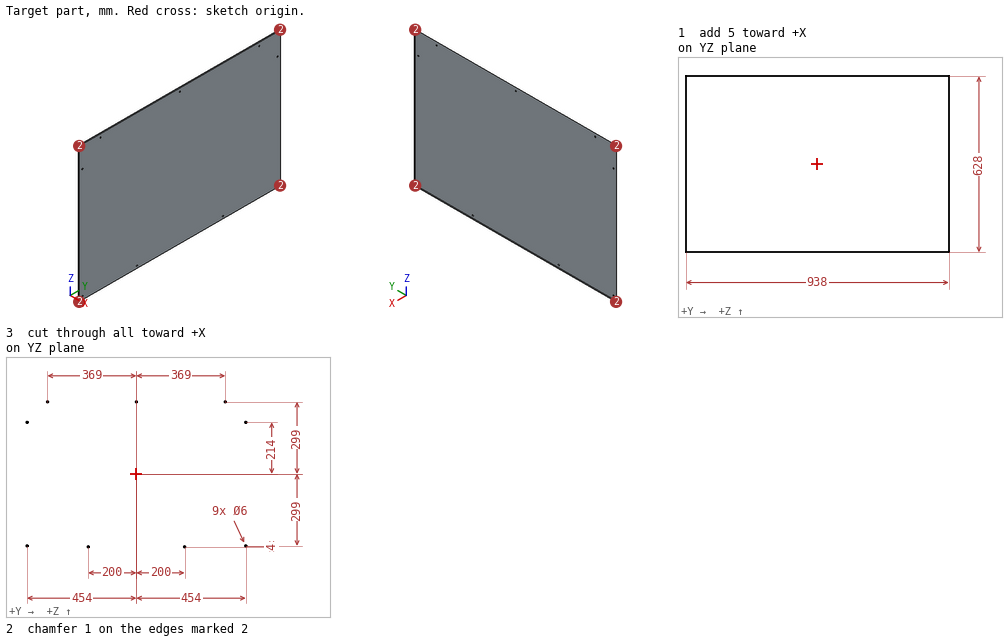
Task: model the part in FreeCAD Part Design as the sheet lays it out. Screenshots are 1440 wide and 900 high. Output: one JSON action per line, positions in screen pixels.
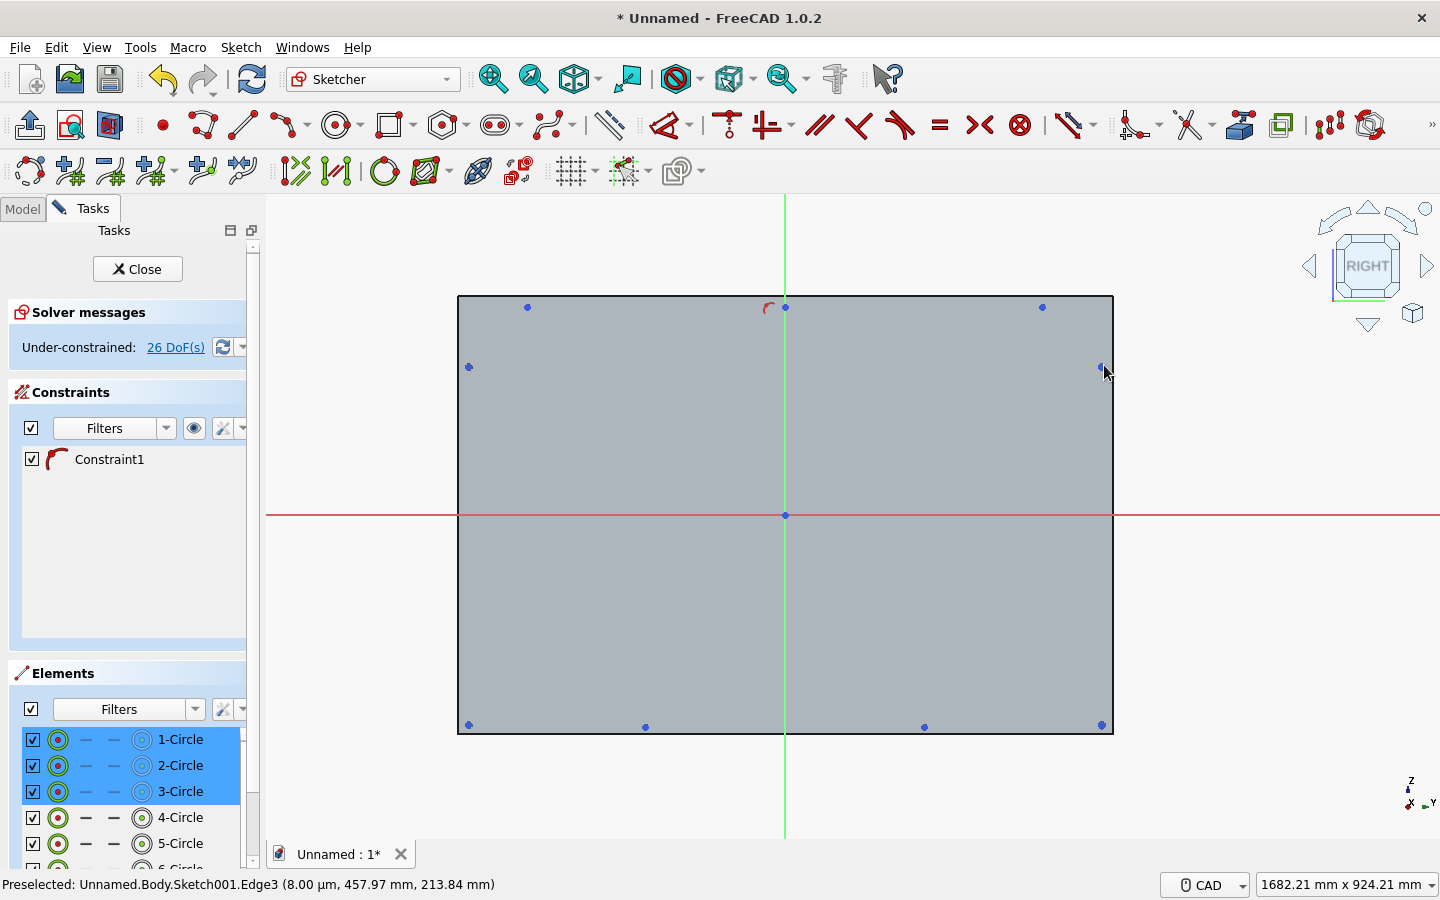
{"action": "scroll", "coordinate": [1045, 305], "scroll_direction": "up", "scroll_amount": 9}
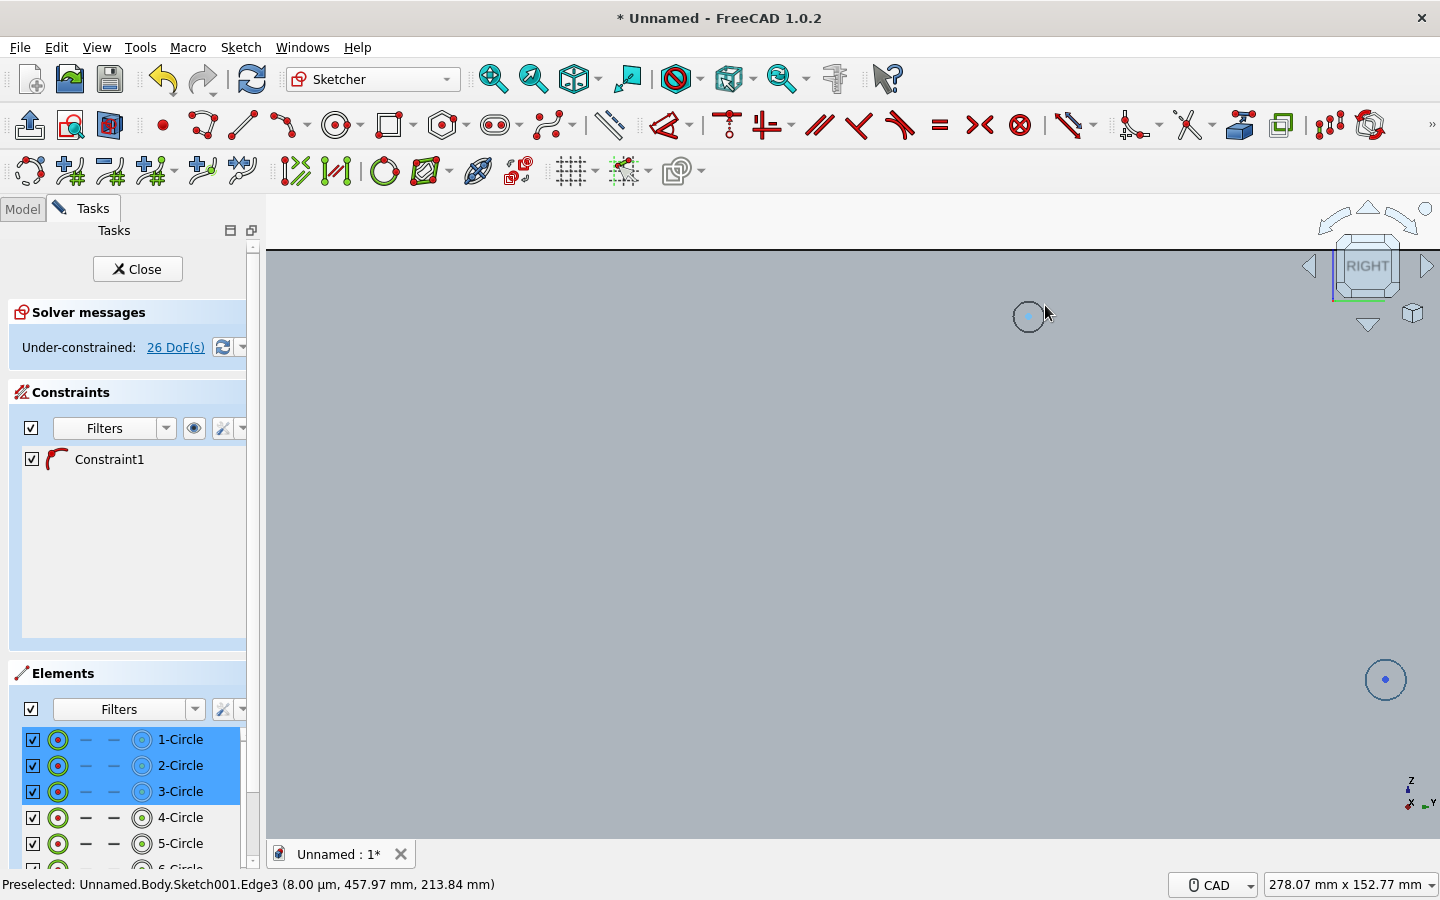
{"action": "left_click", "coordinate": [1040, 306]}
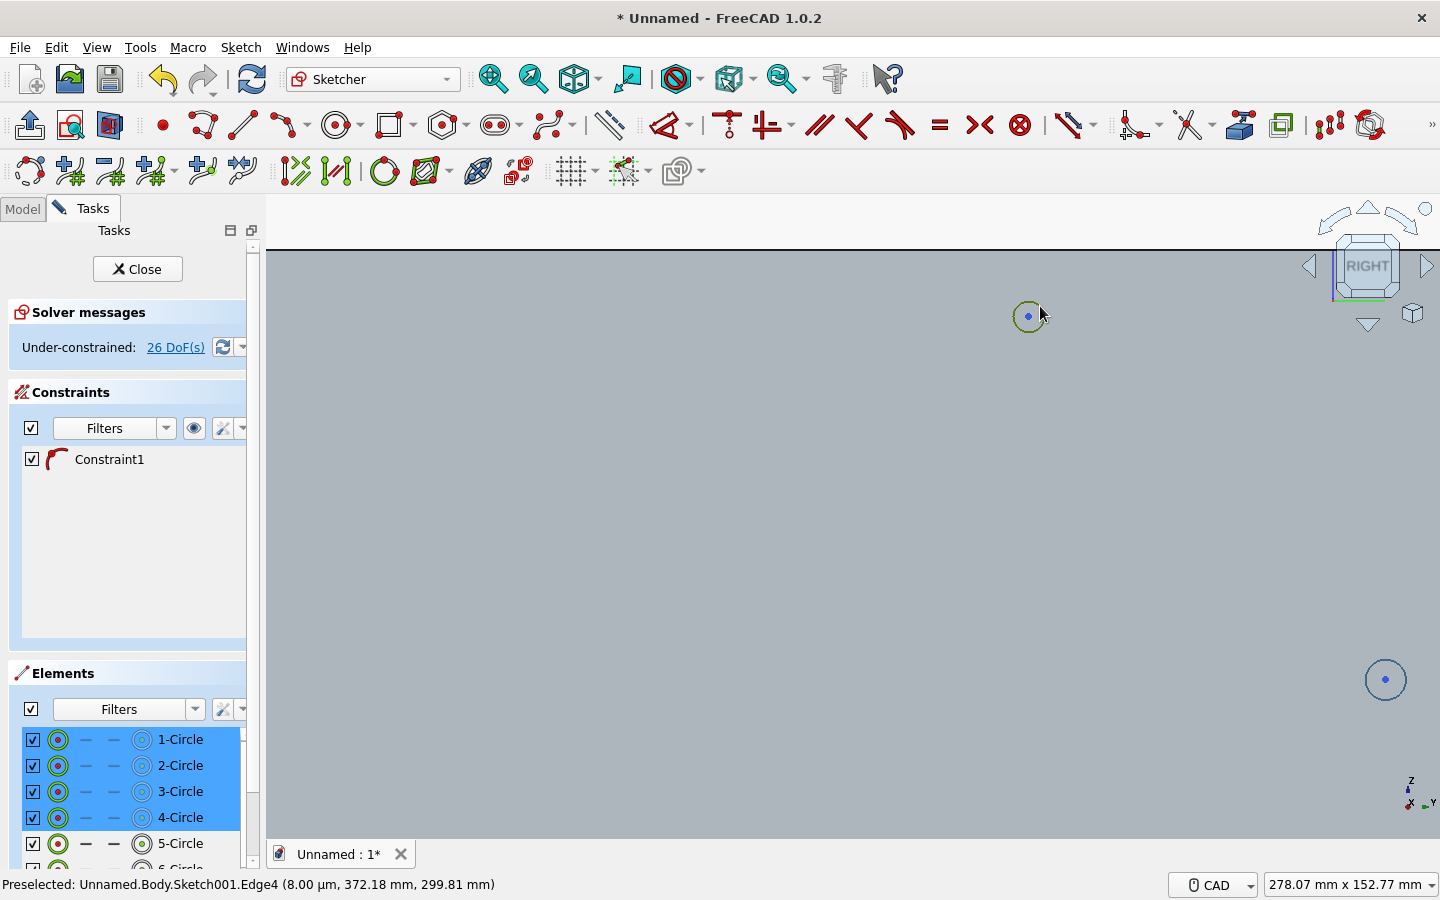
{"action": "scroll", "coordinate": [1045, 305], "scroll_direction": "down", "scroll_amount": 9}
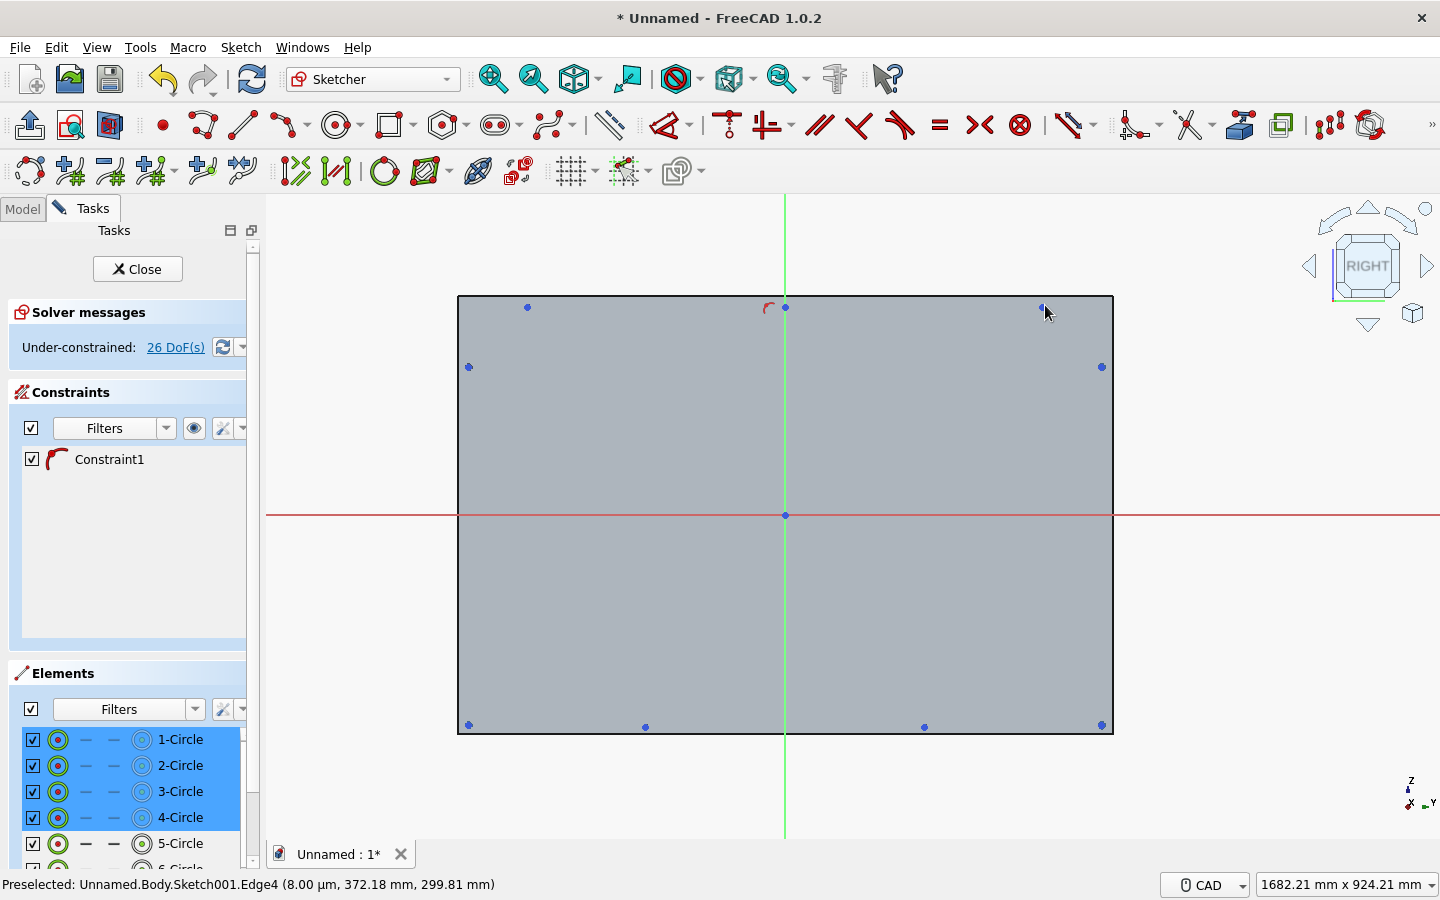
{"action": "scroll", "coordinate": [530, 305], "scroll_direction": "up", "scroll_amount": 9}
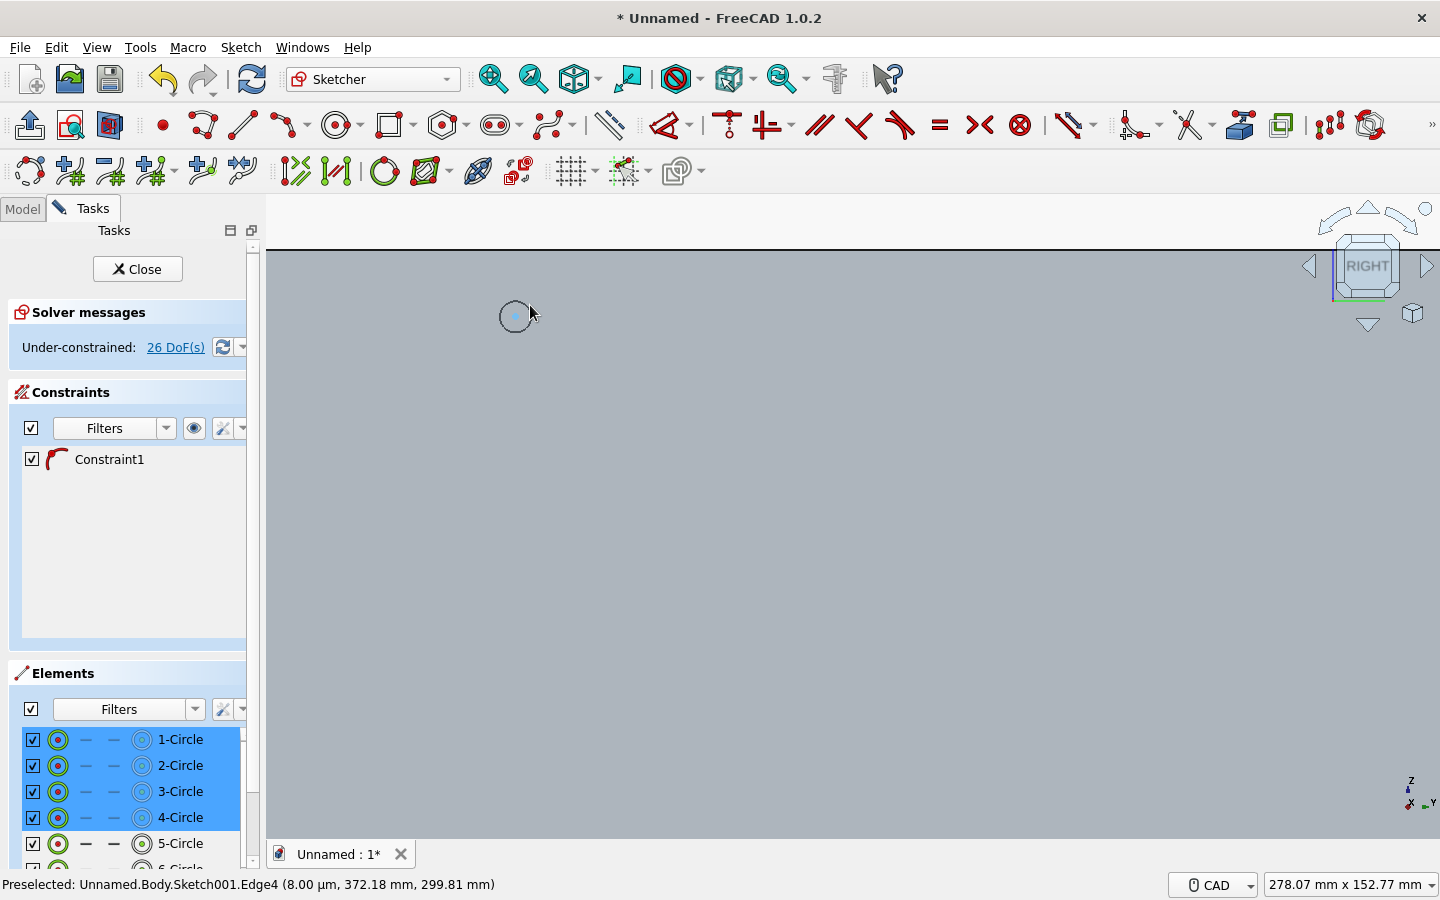
{"action": "left_click", "coordinate": [527, 306]}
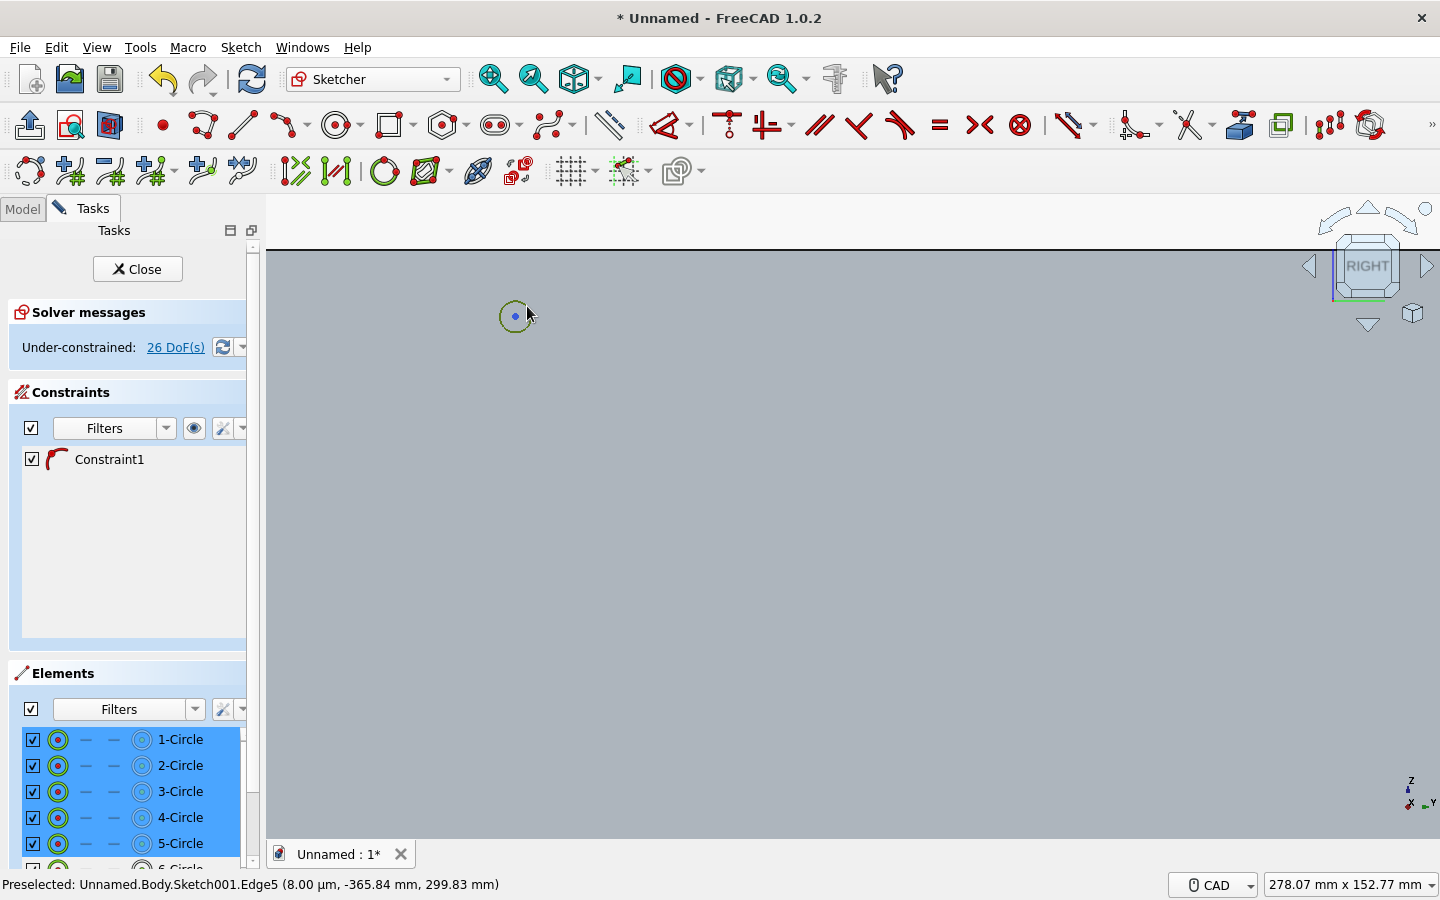
{"action": "scroll", "coordinate": [529, 305], "scroll_direction": "down", "scroll_amount": 9}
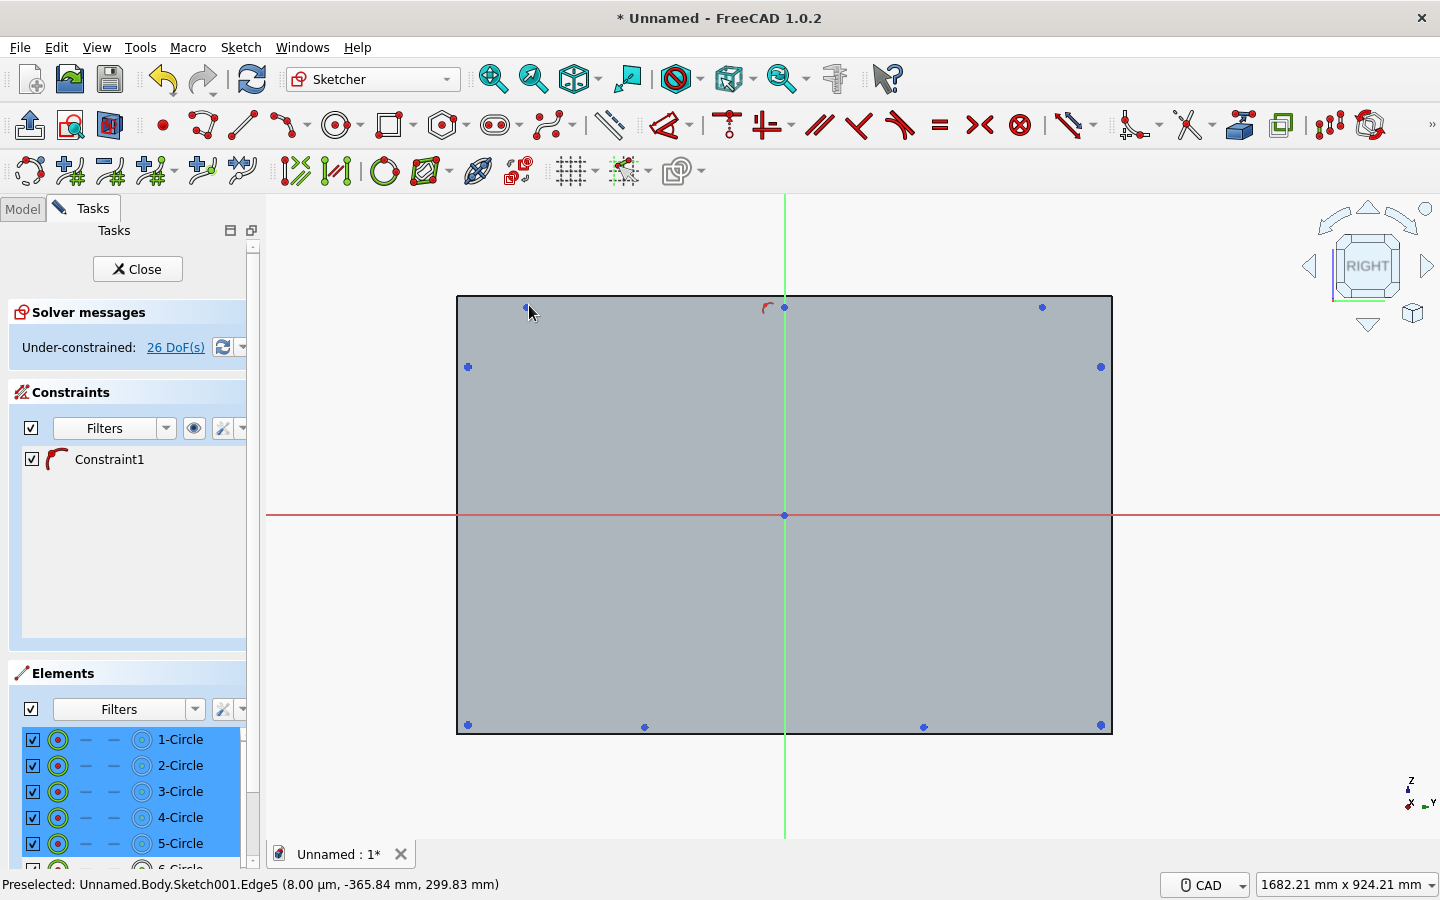
{"action": "scroll", "coordinate": [470, 365], "scroll_direction": "up", "scroll_amount": 8}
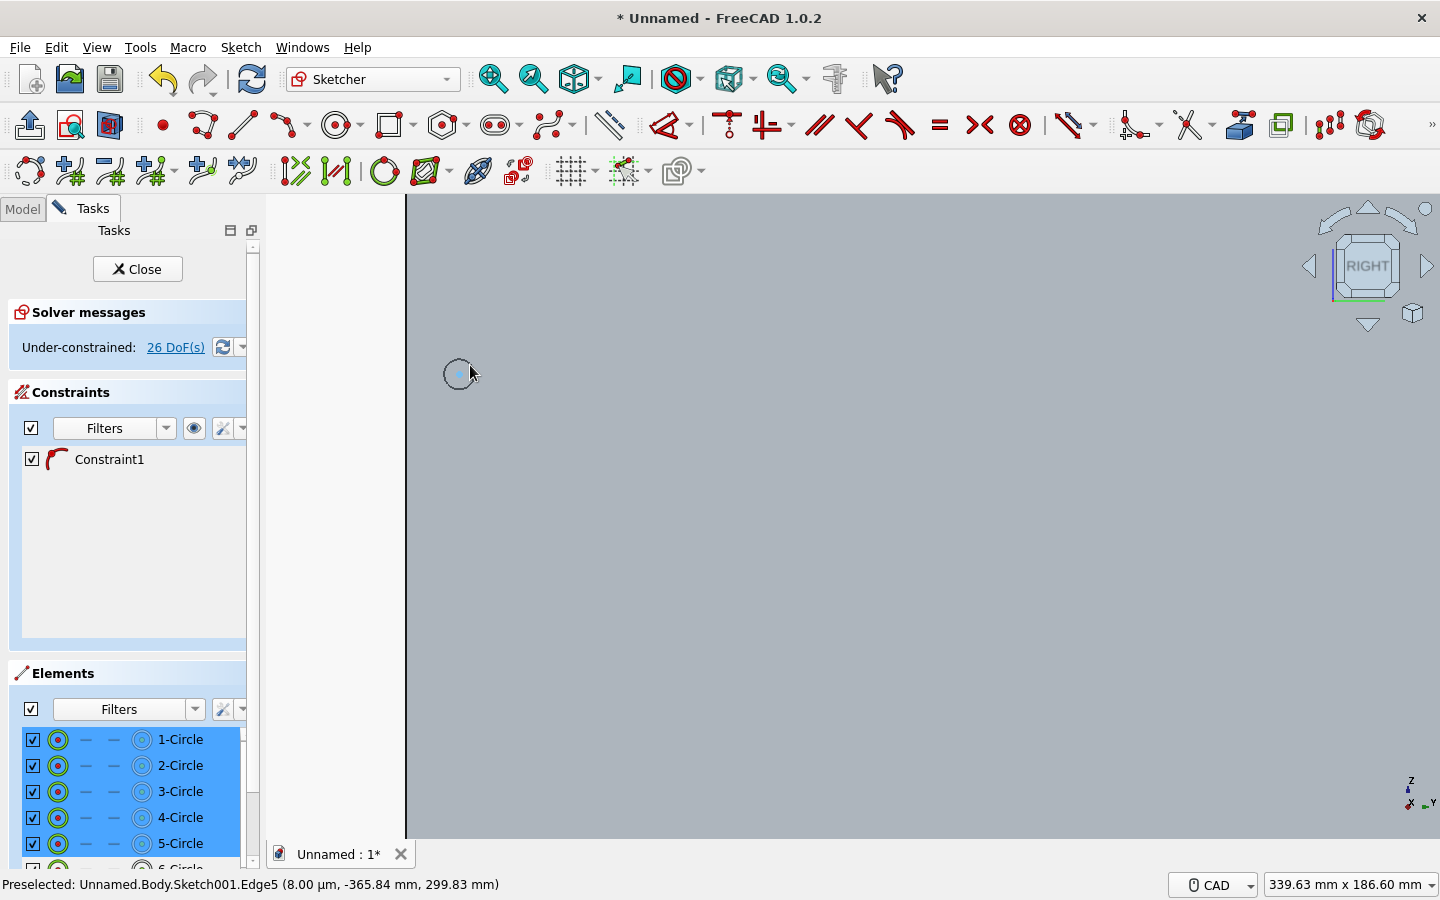
{"action": "left_click", "coordinate": [470, 364]}